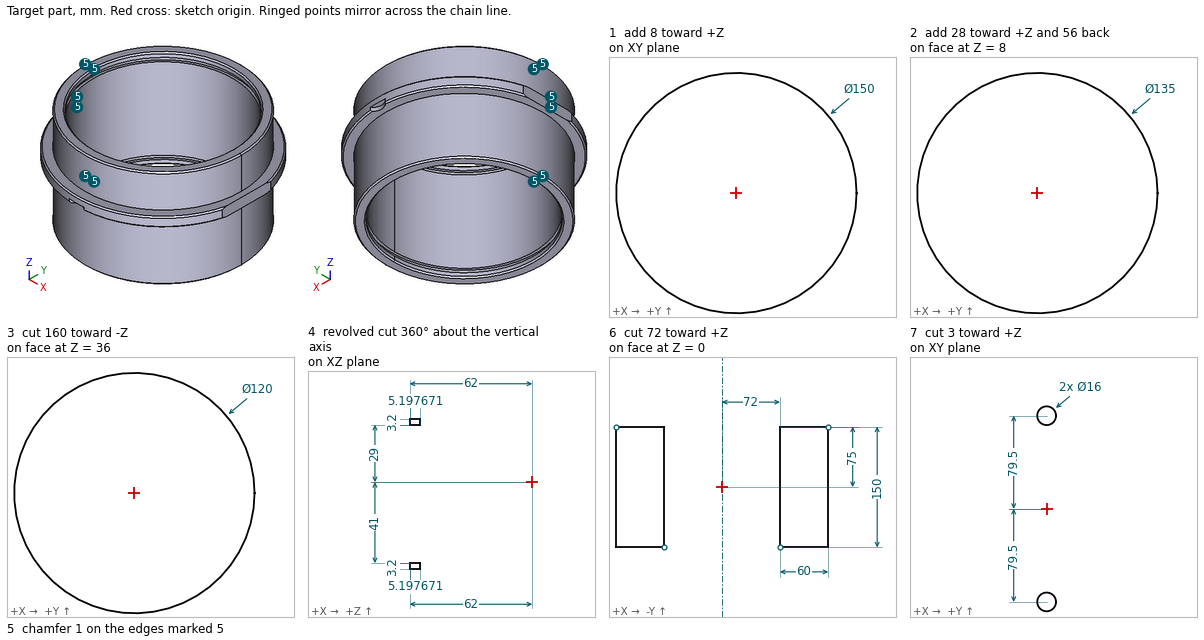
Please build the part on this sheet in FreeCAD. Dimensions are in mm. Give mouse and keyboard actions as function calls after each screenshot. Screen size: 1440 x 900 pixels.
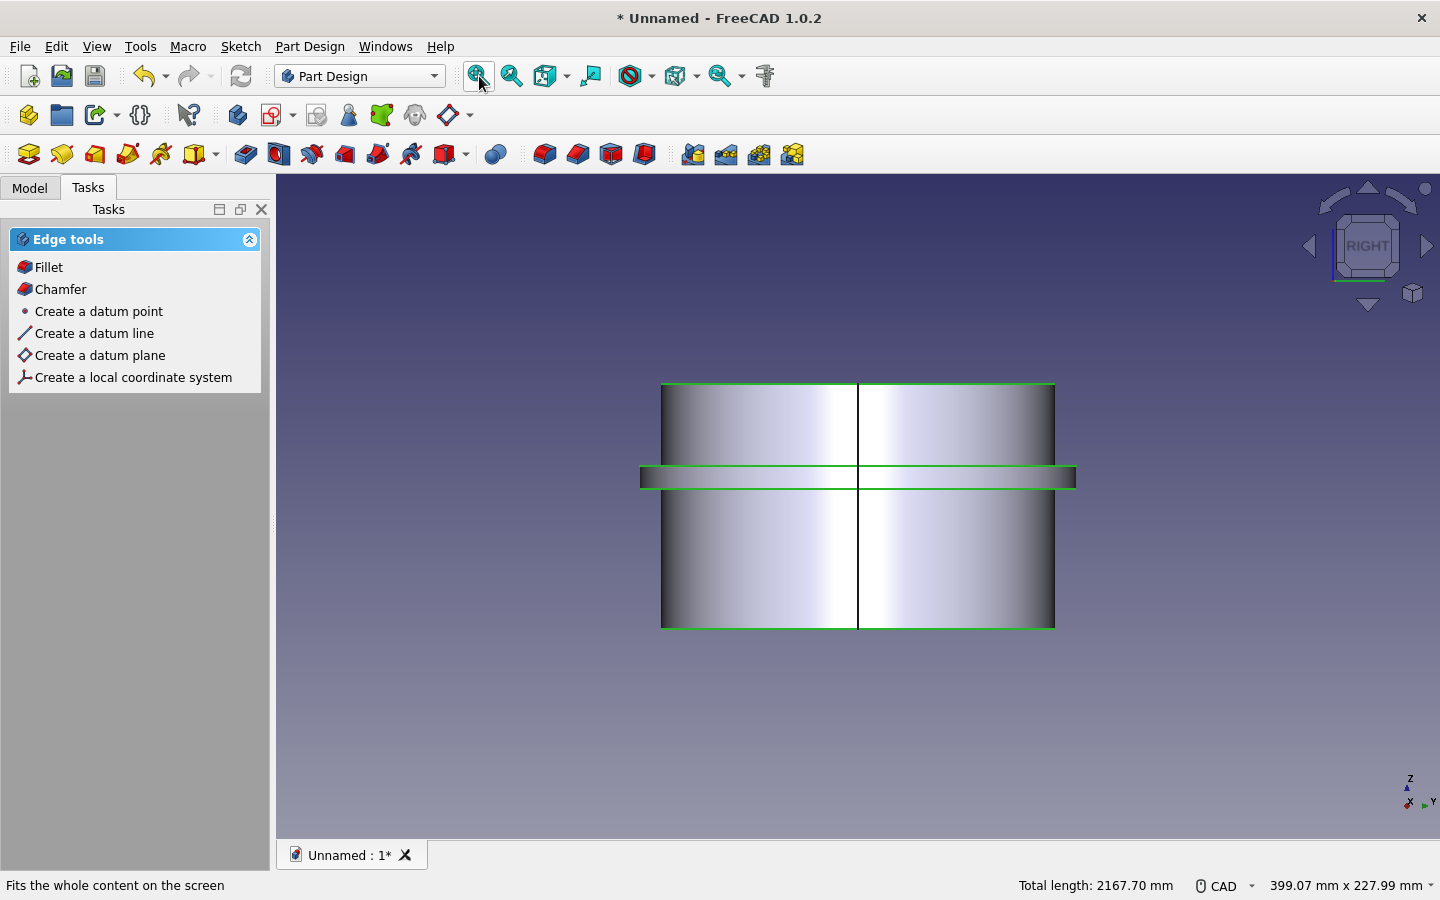
key(5)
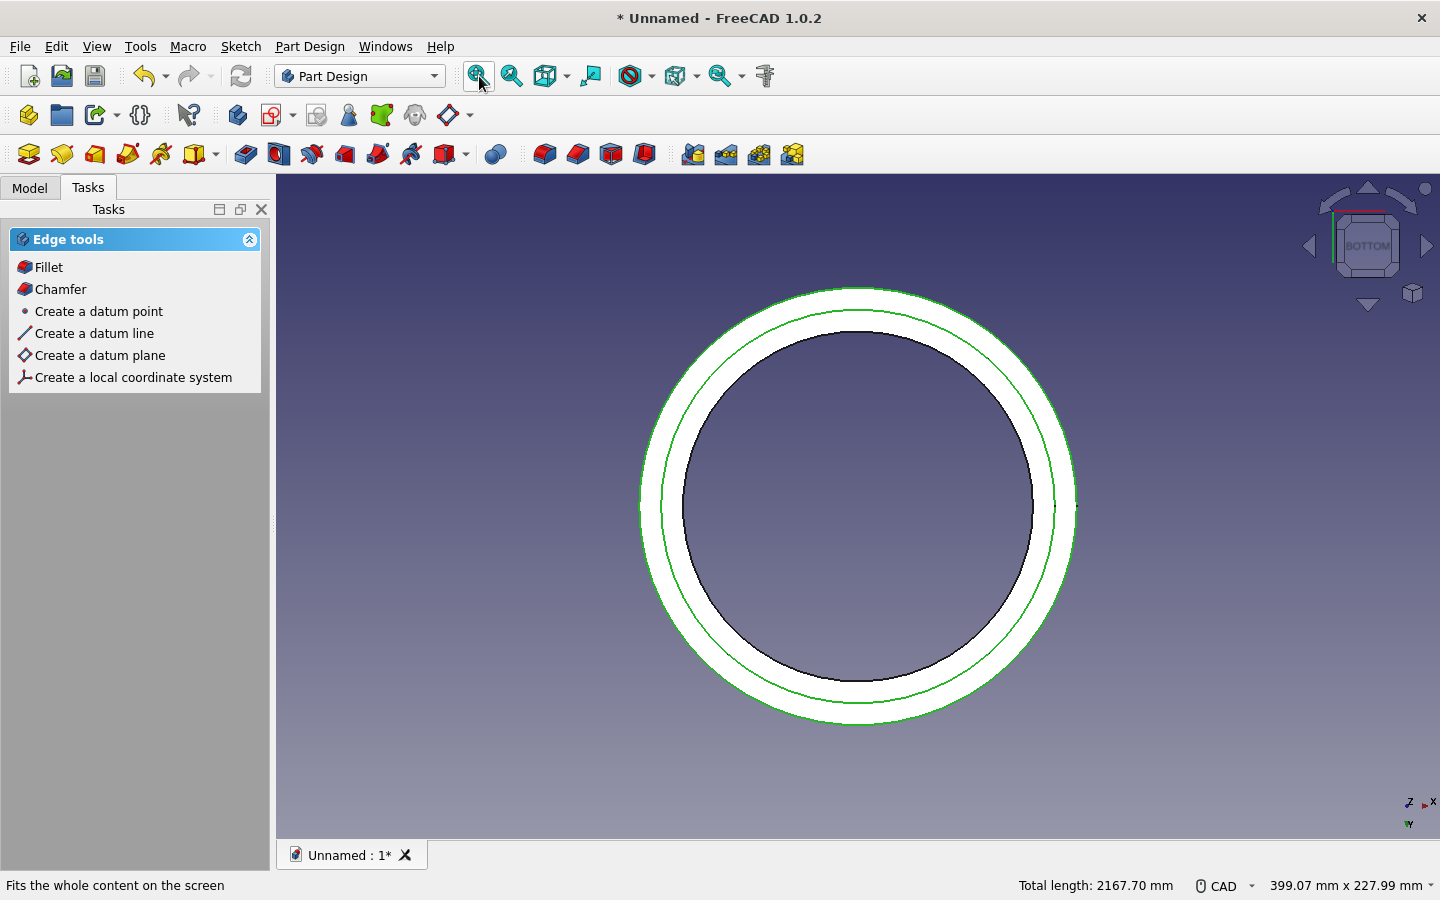
click(683, 505, ctrl)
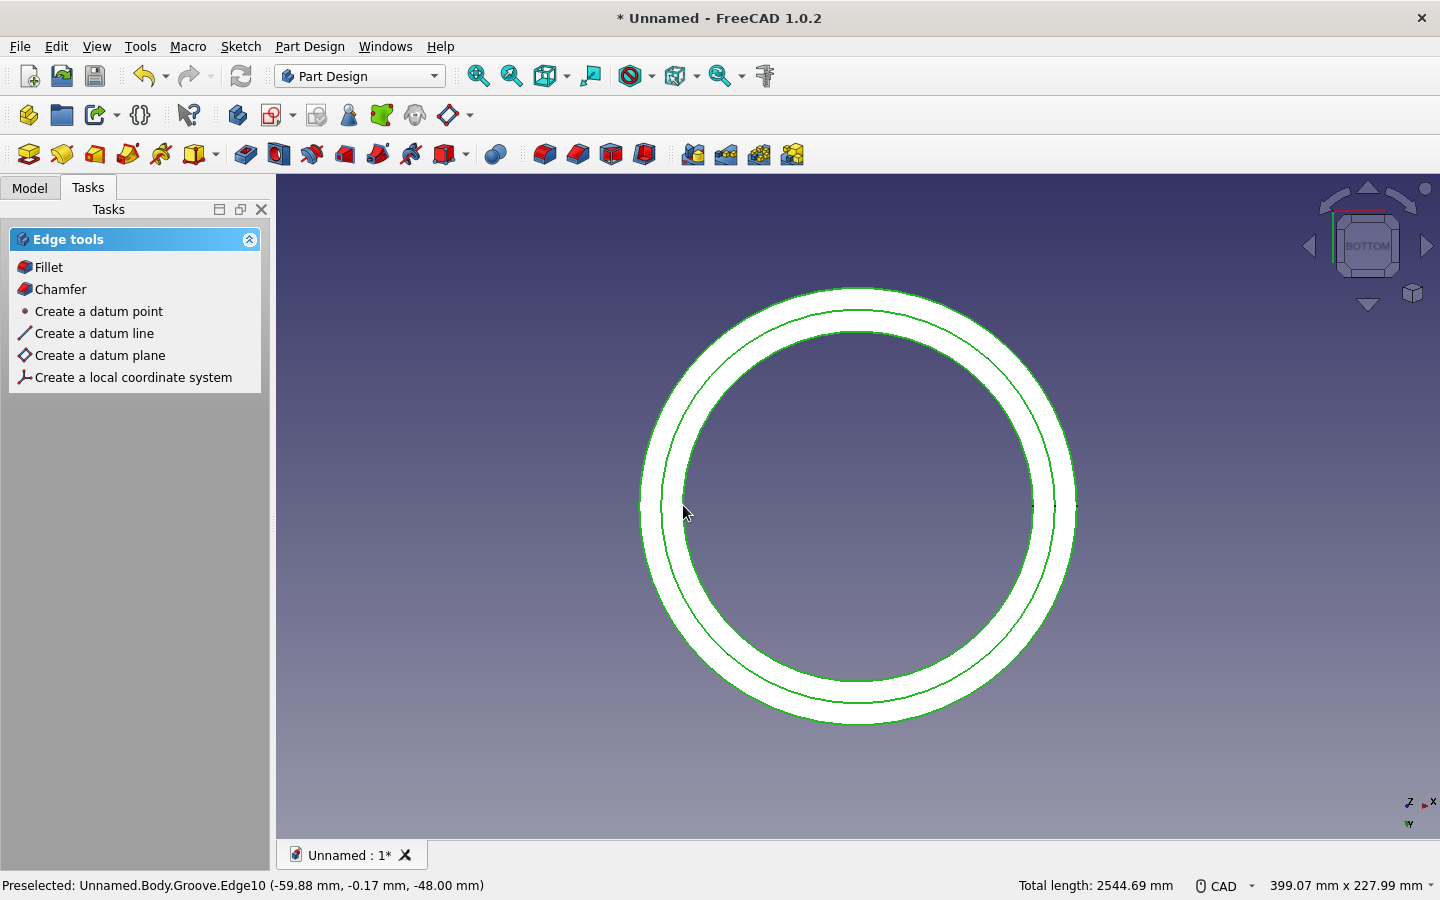
click(578, 154)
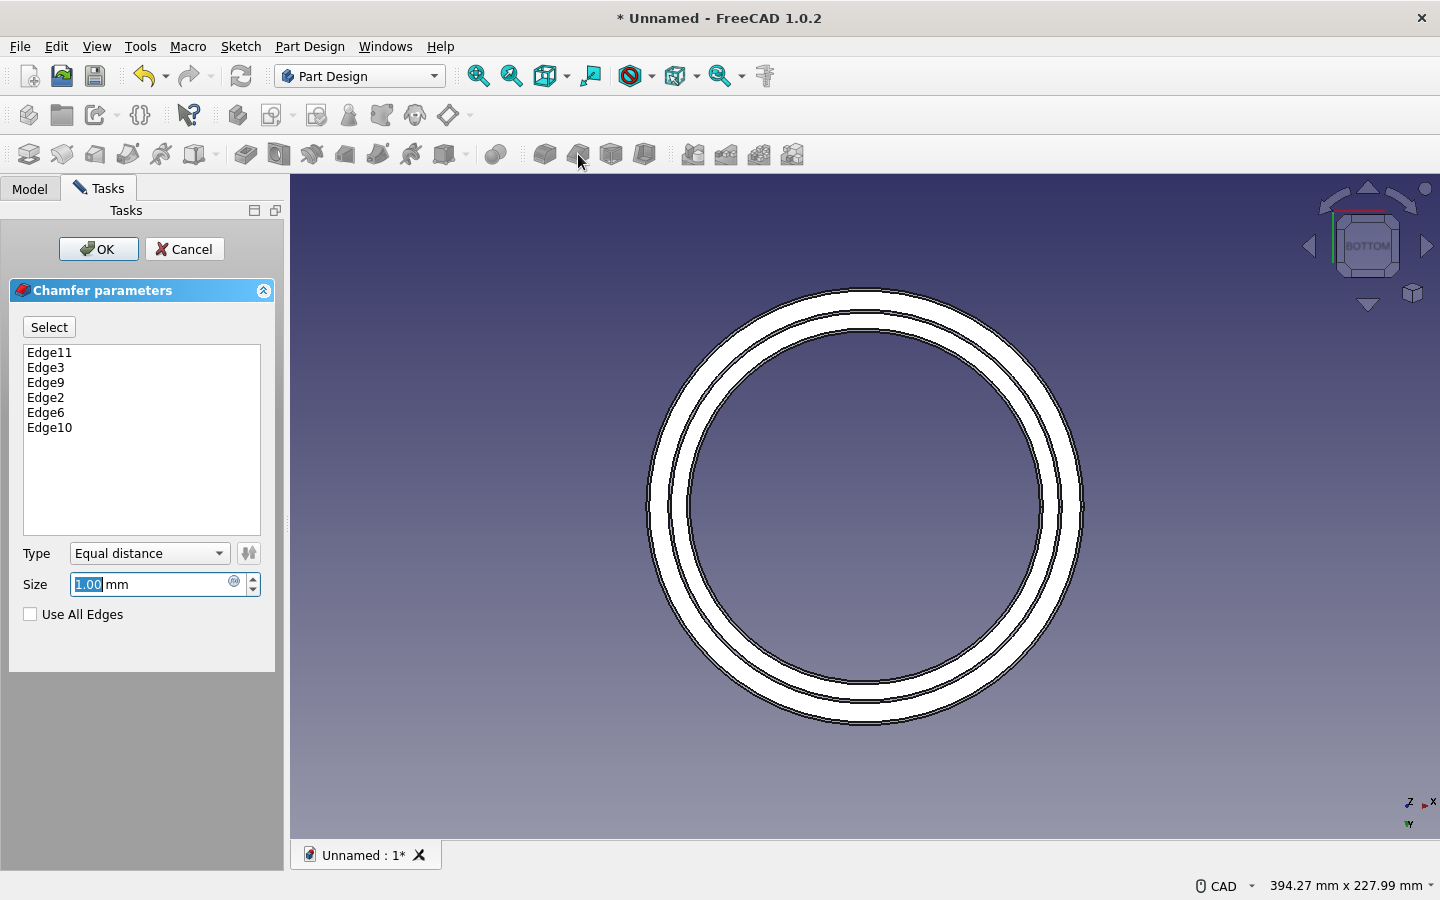
text(1)
key(Tab)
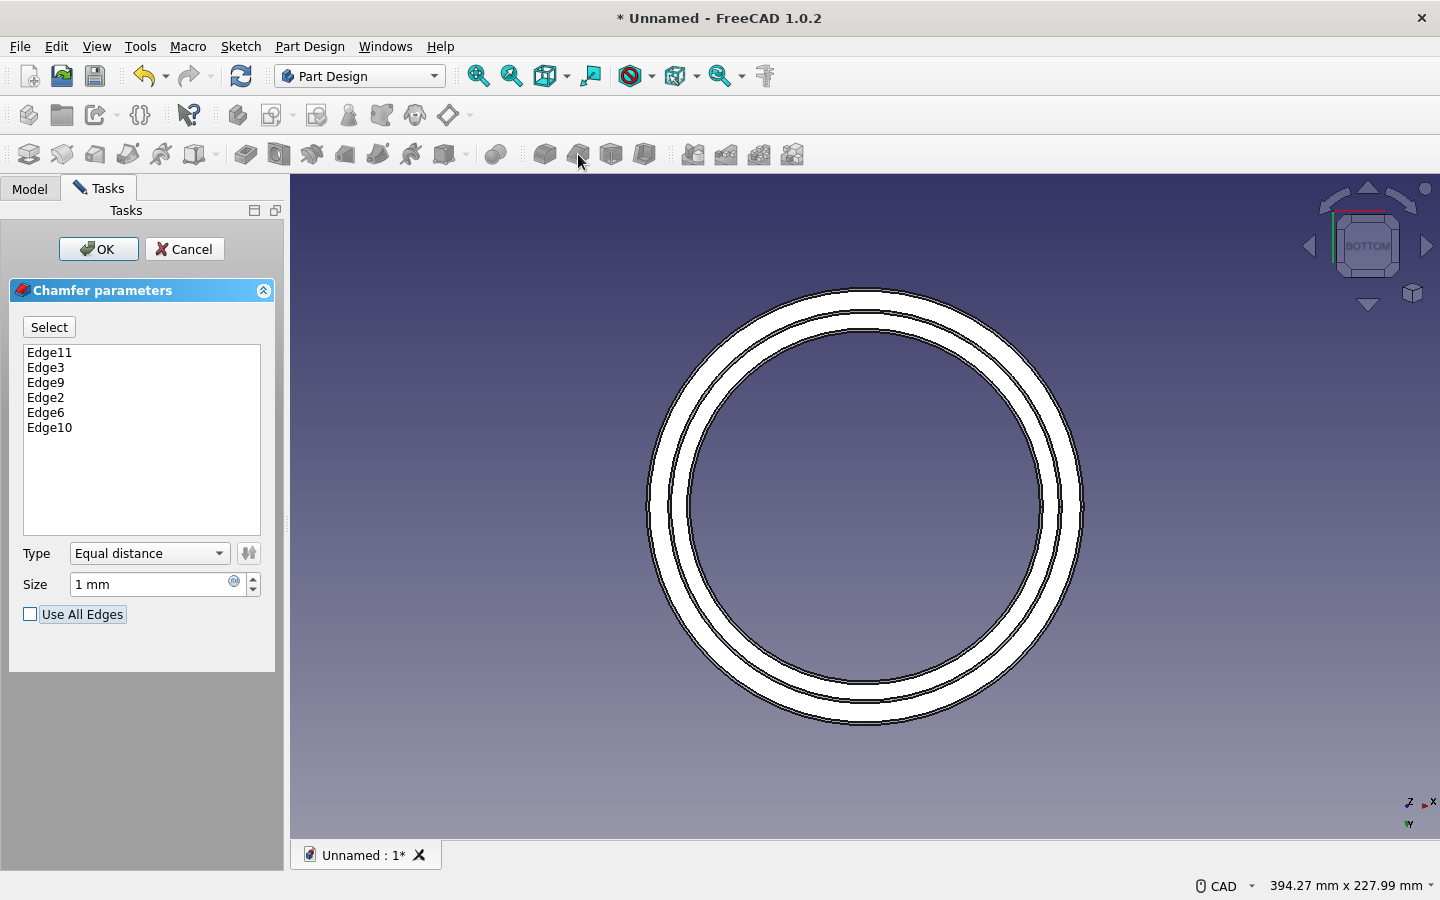
click(99, 249)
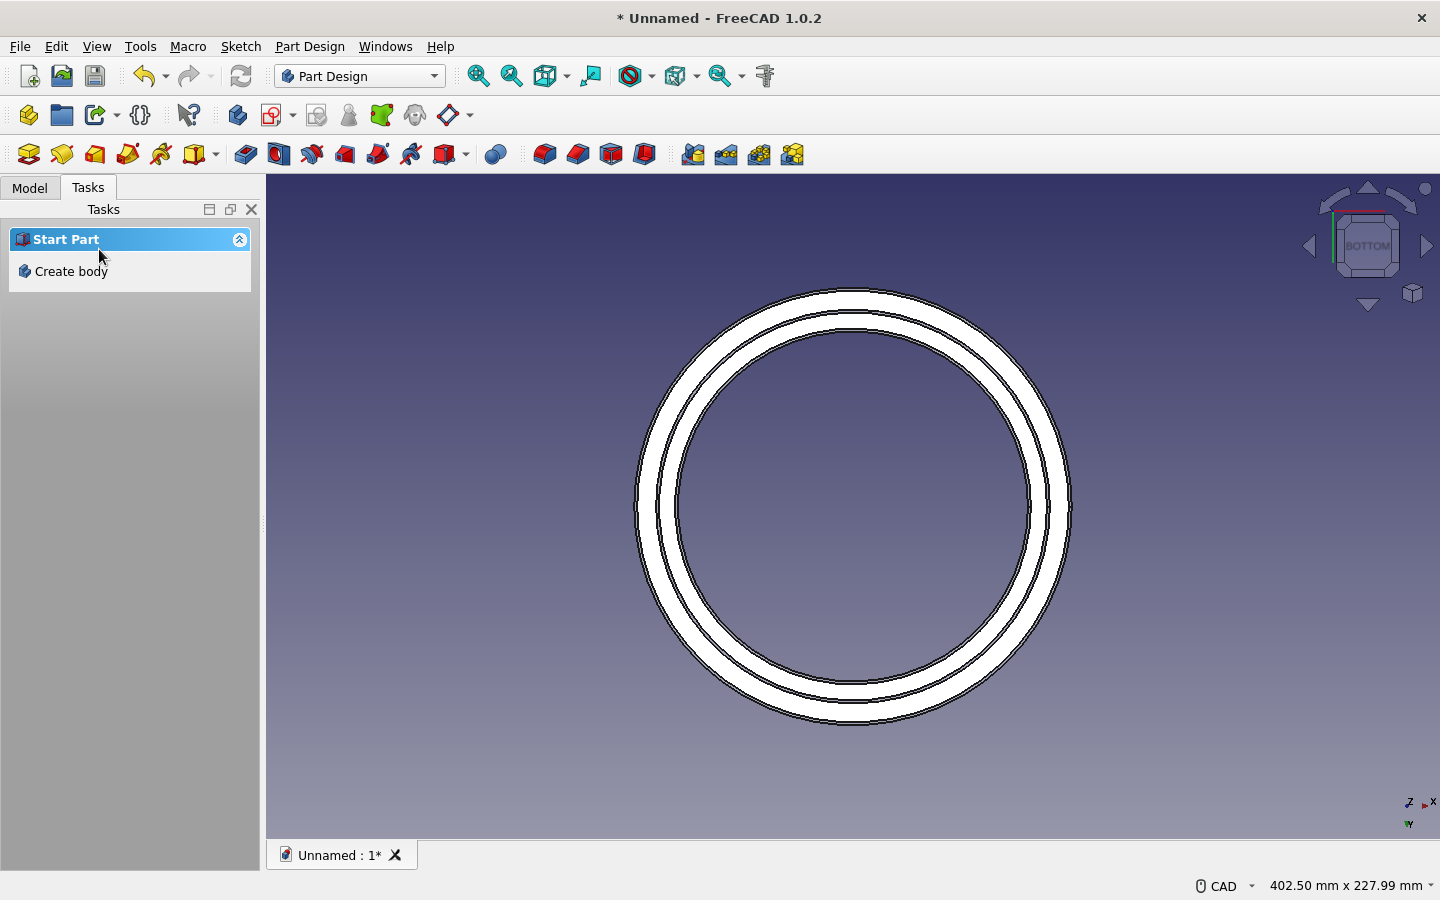
scroll(978, 673, up, 4)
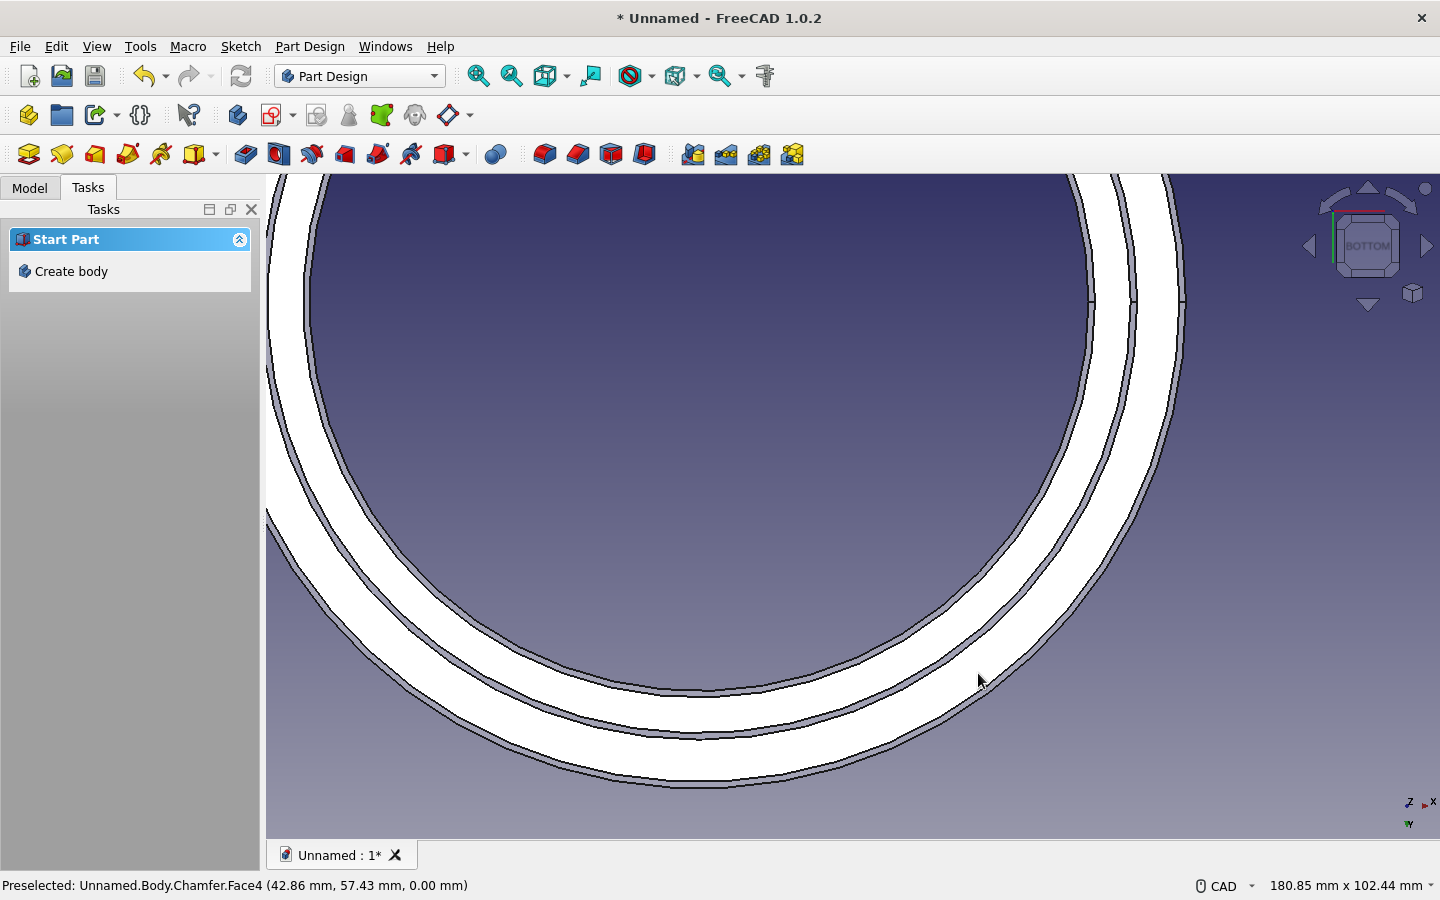
click(978, 674)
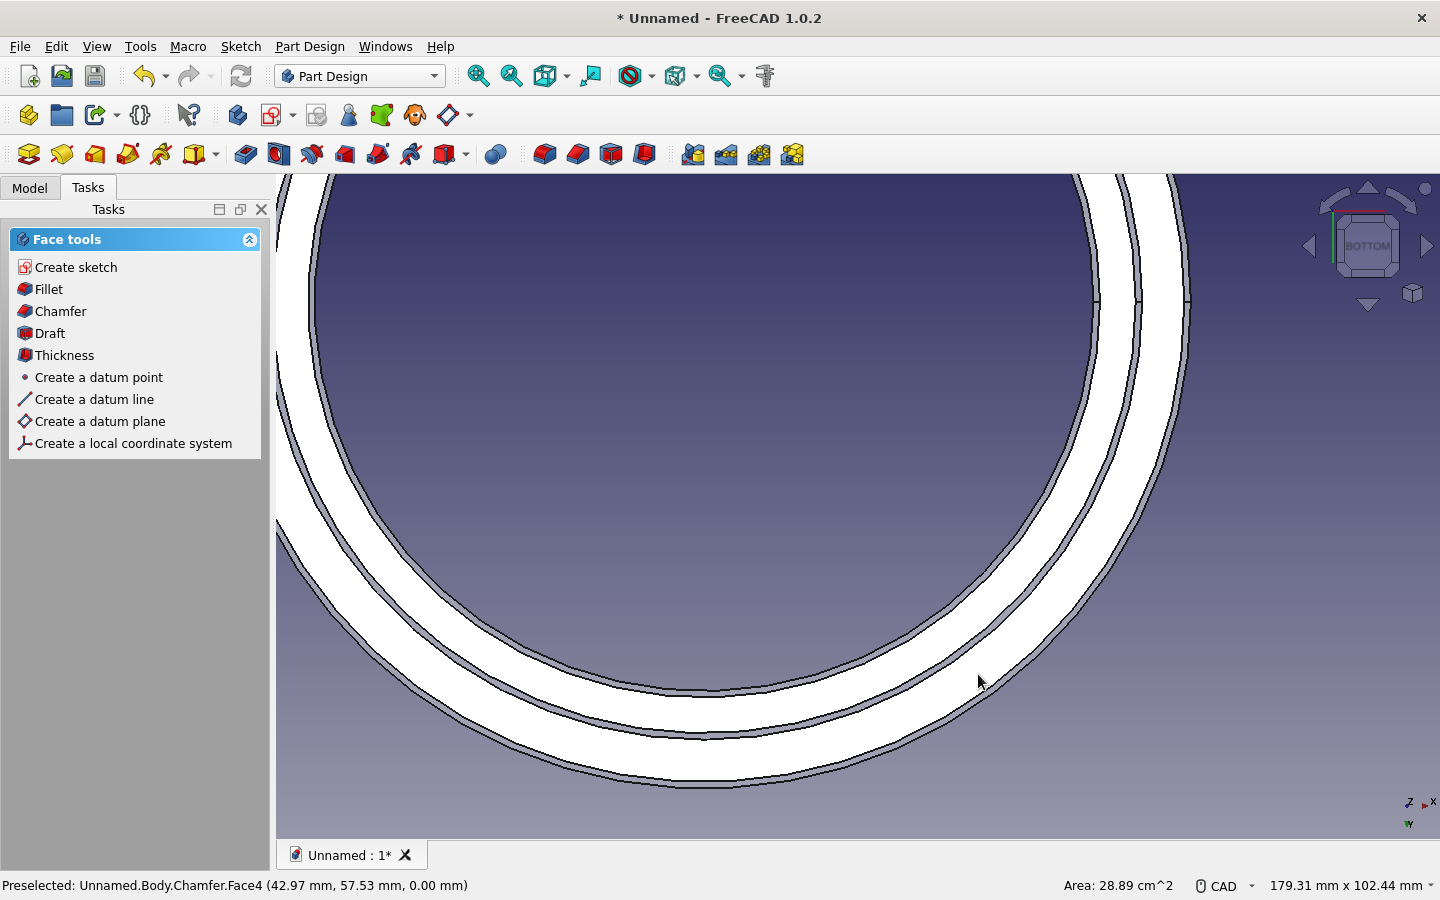
click(270, 116)